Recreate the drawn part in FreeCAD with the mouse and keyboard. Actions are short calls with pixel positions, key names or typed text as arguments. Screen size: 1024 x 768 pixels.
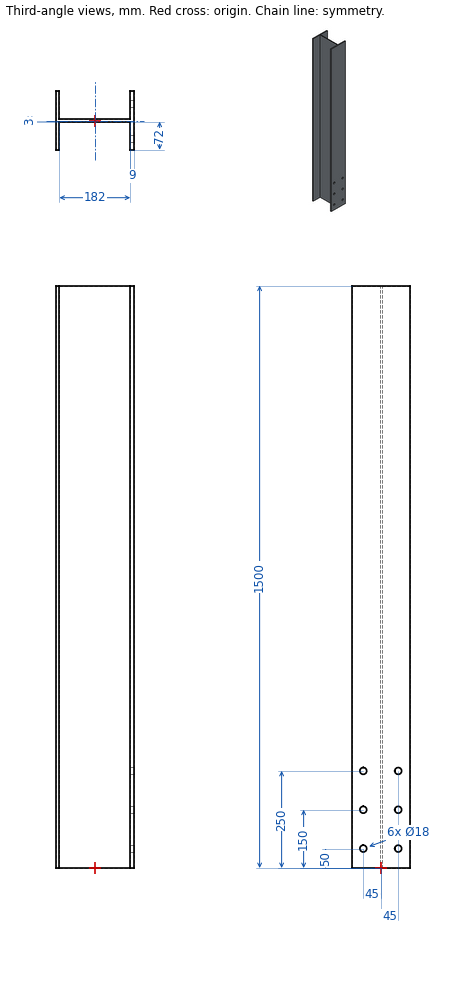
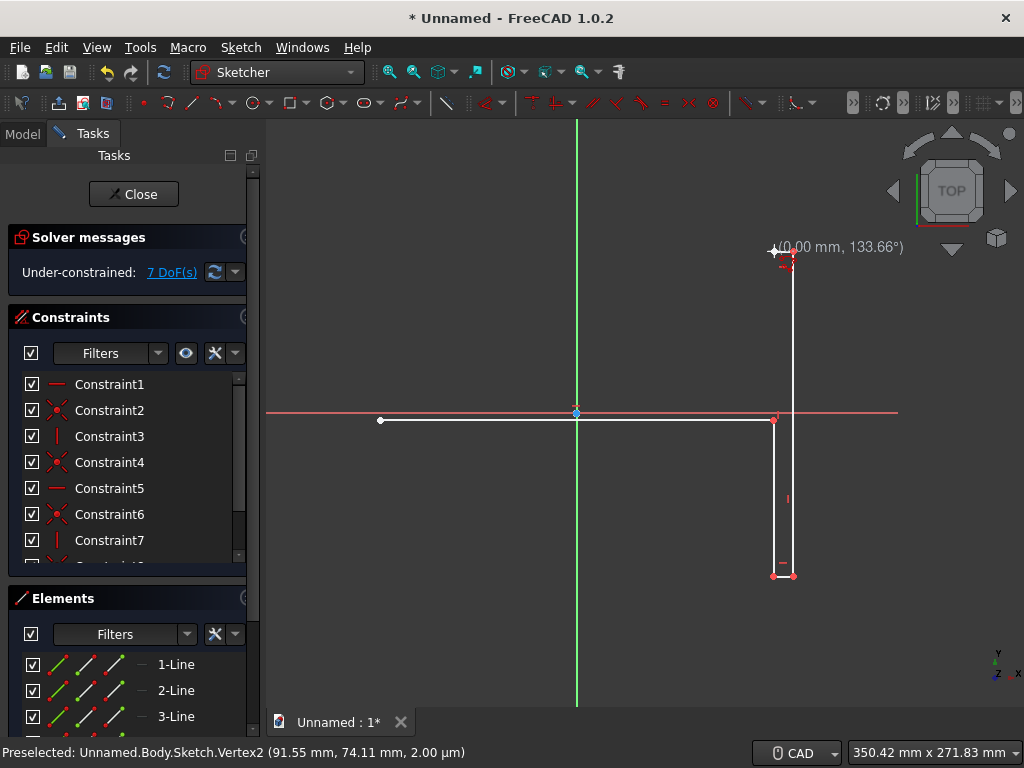
scroll(774, 407, up, 5)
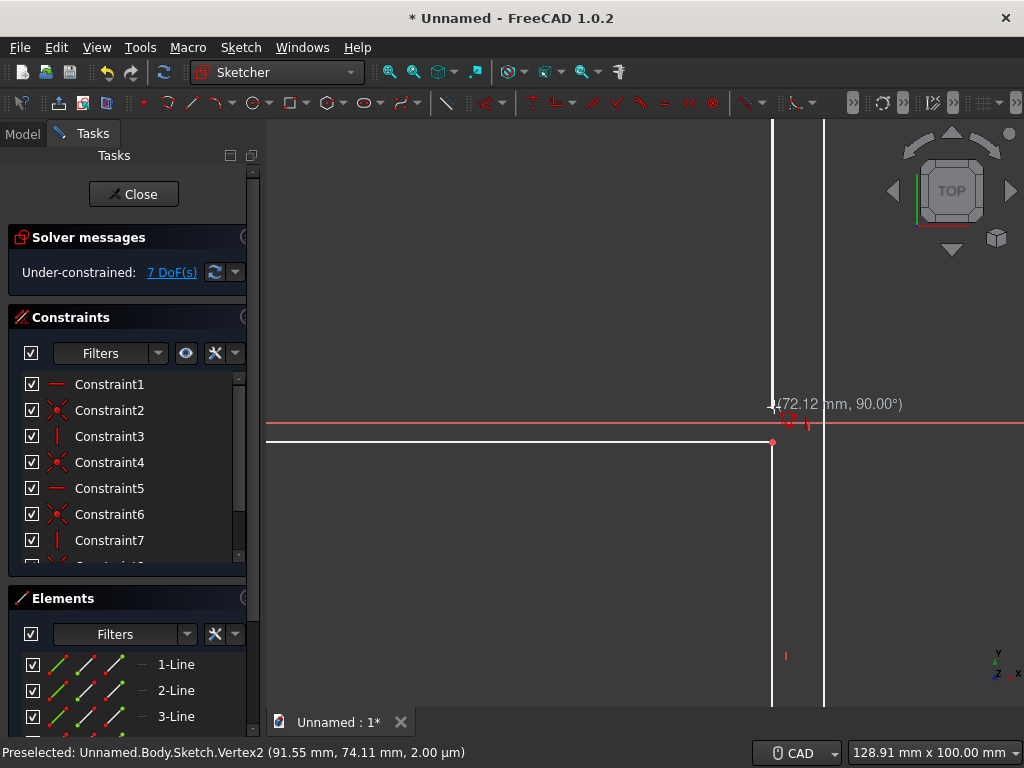
click(773, 406)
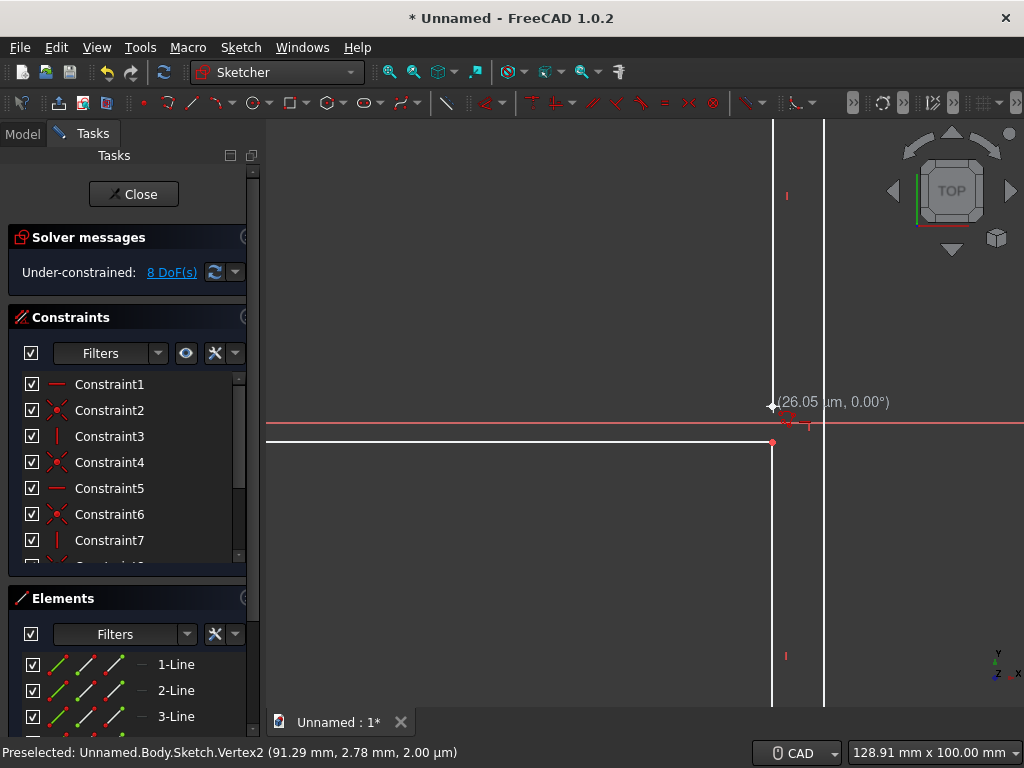
scroll(774, 407, down, 5)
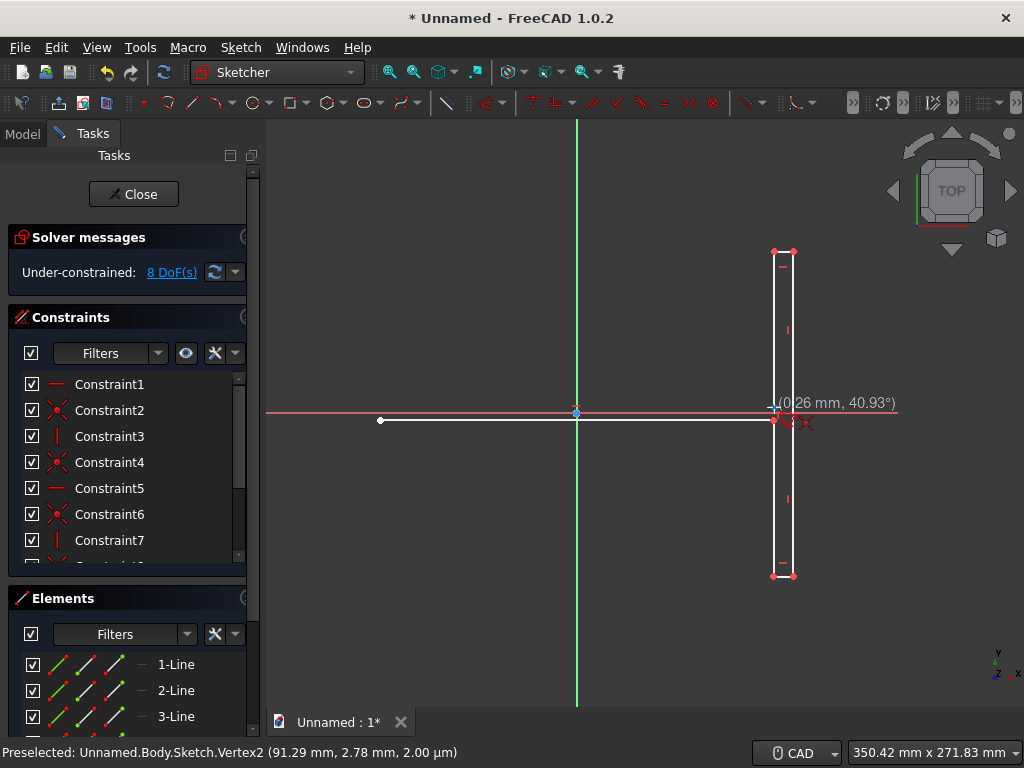
scroll(380, 407, up, 5)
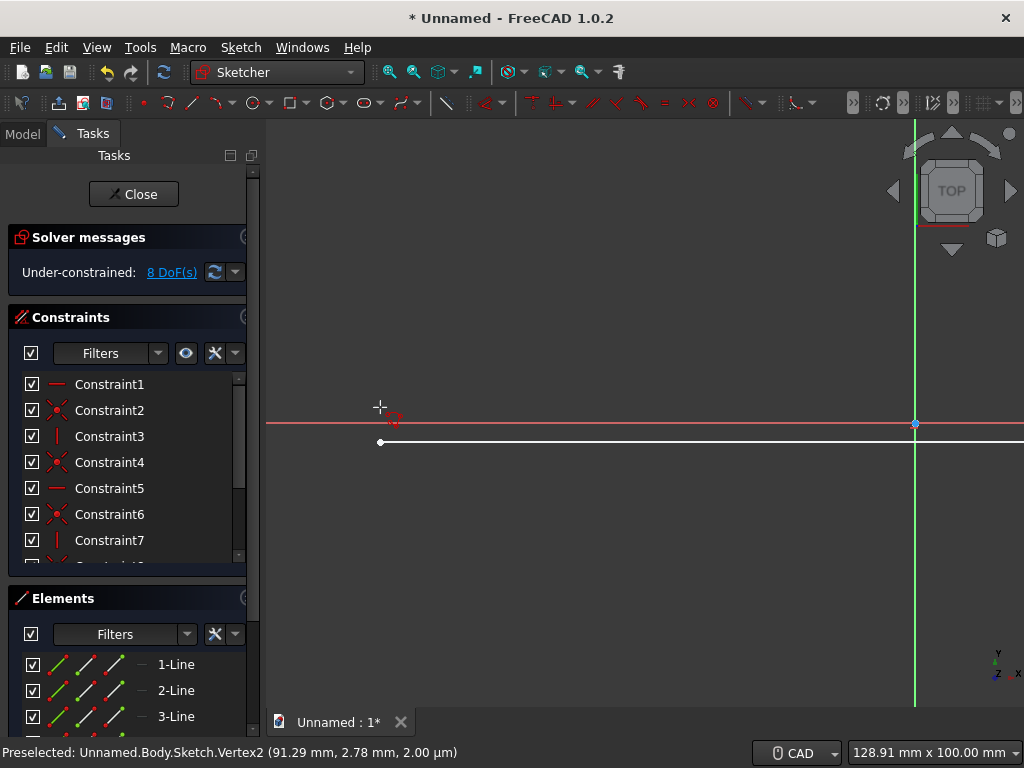
click(380, 406)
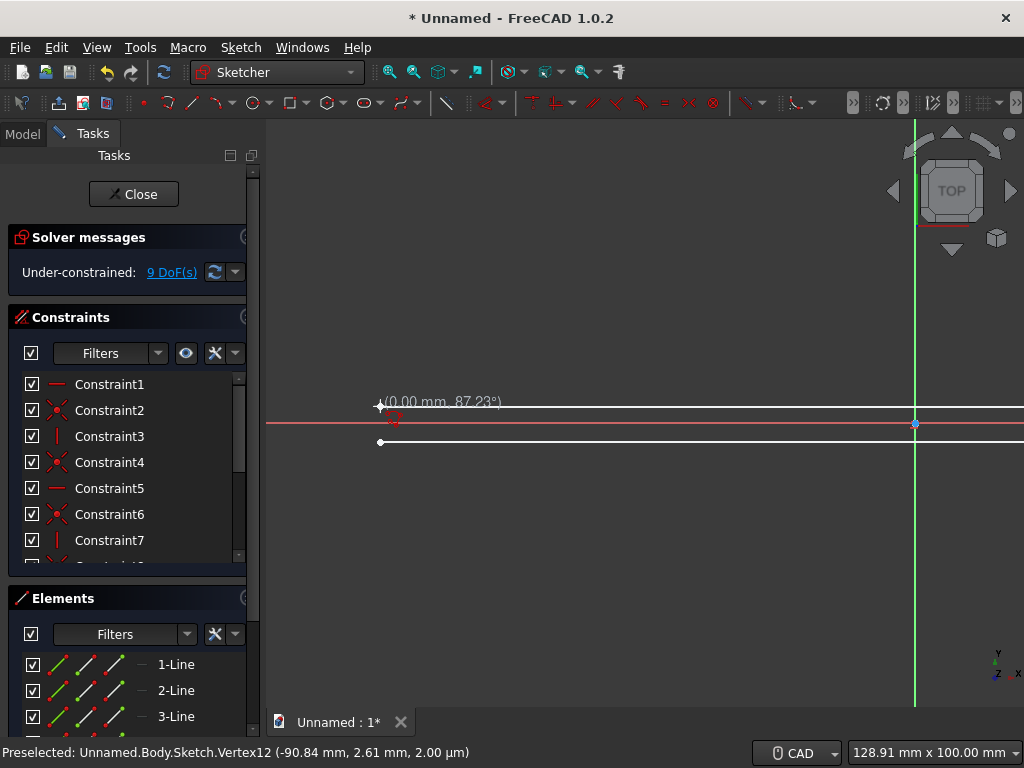
scroll(379, 407, down, 5)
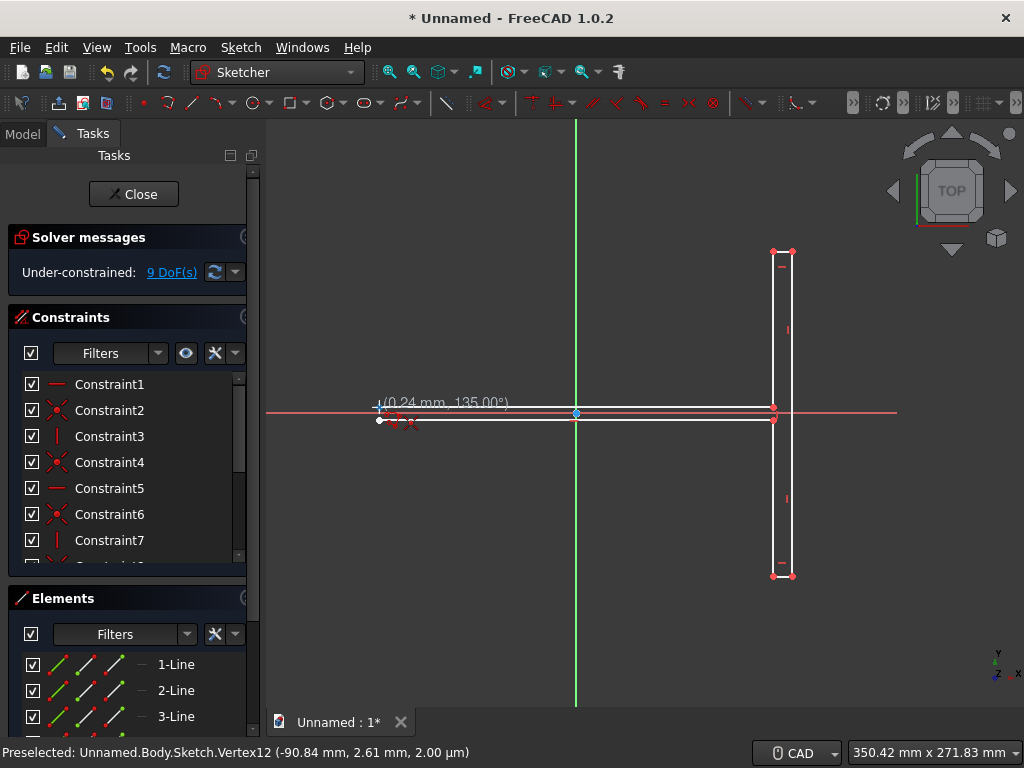
click(379, 251)
click(360, 251)
click(360, 576)
click(379, 576)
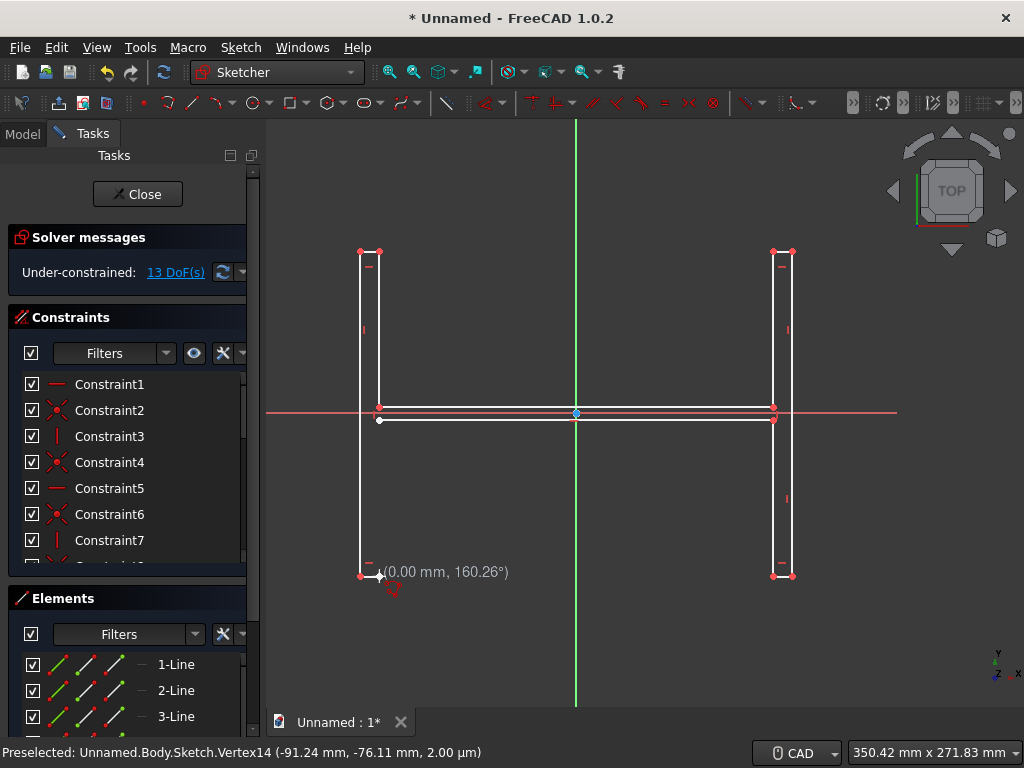
scroll(379, 420, up, 5)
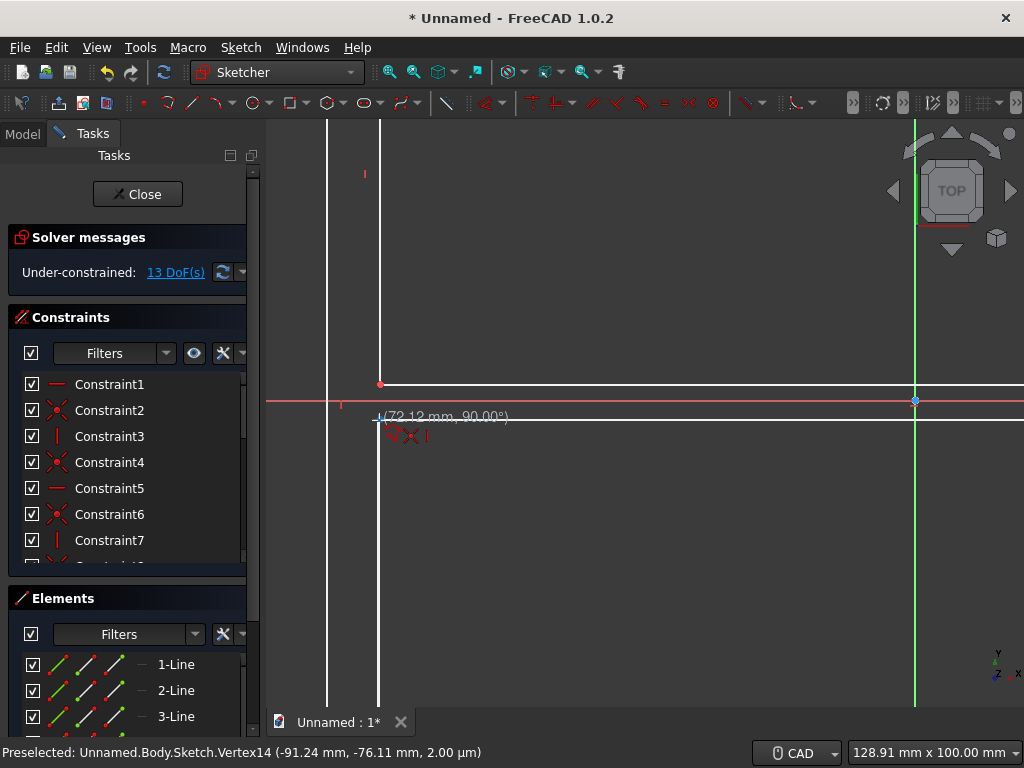
click(380, 420)
key(Escape)
key(Escape)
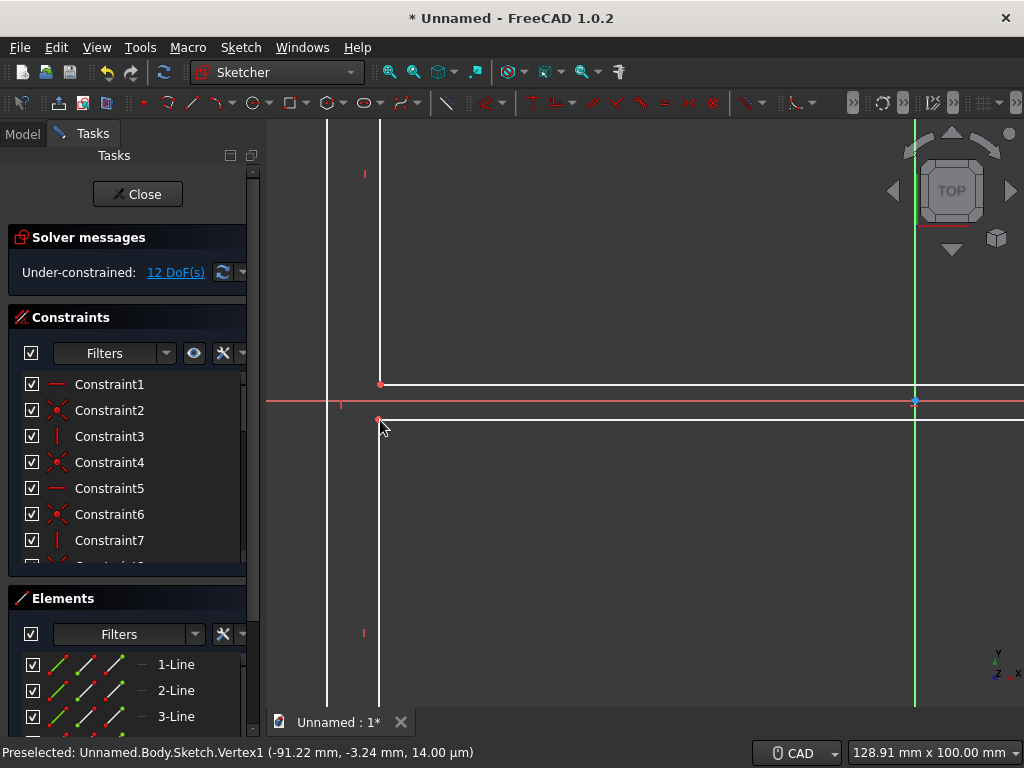
scroll(379, 420, down, 5)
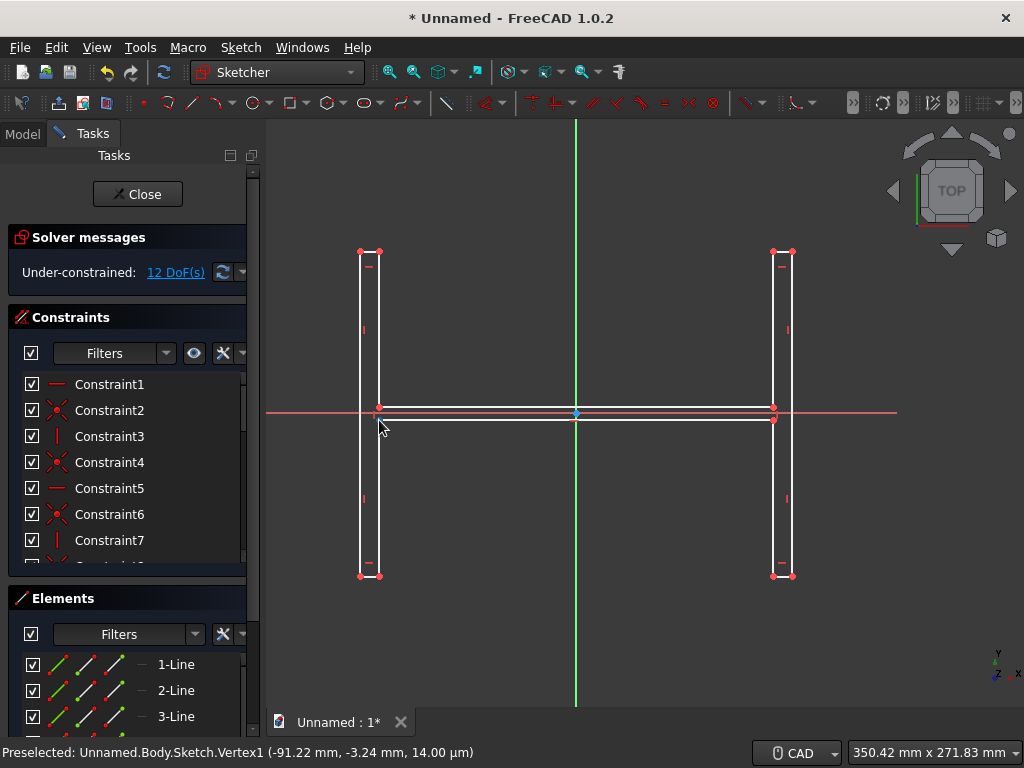
click(773, 577)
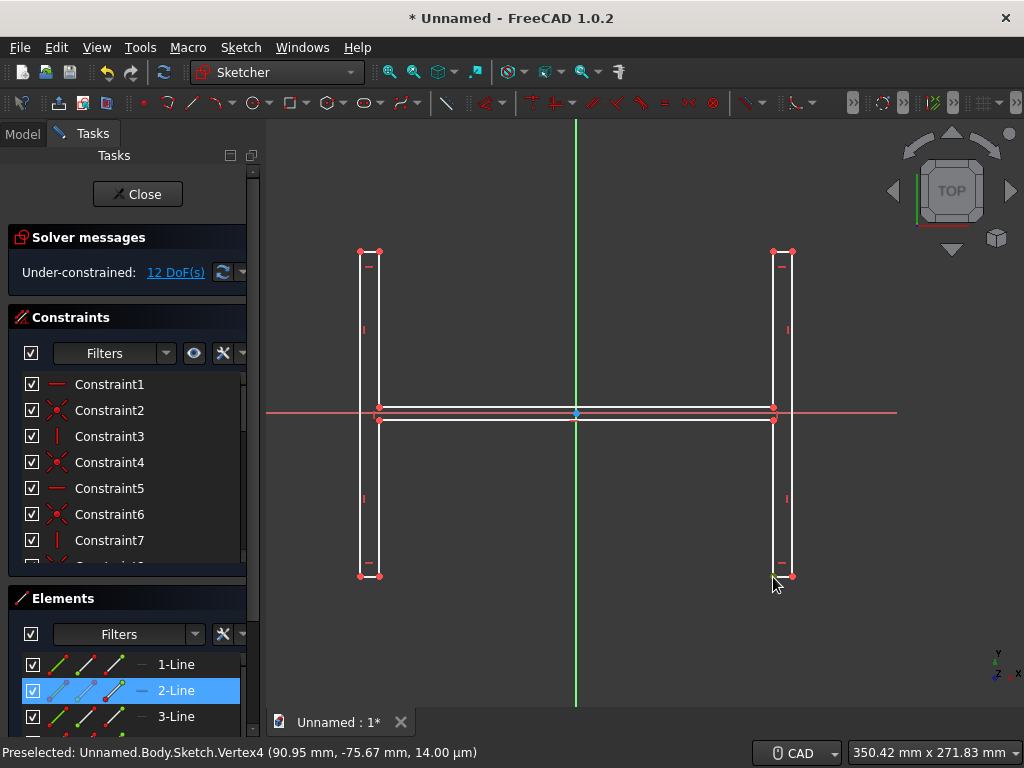
click(773, 252)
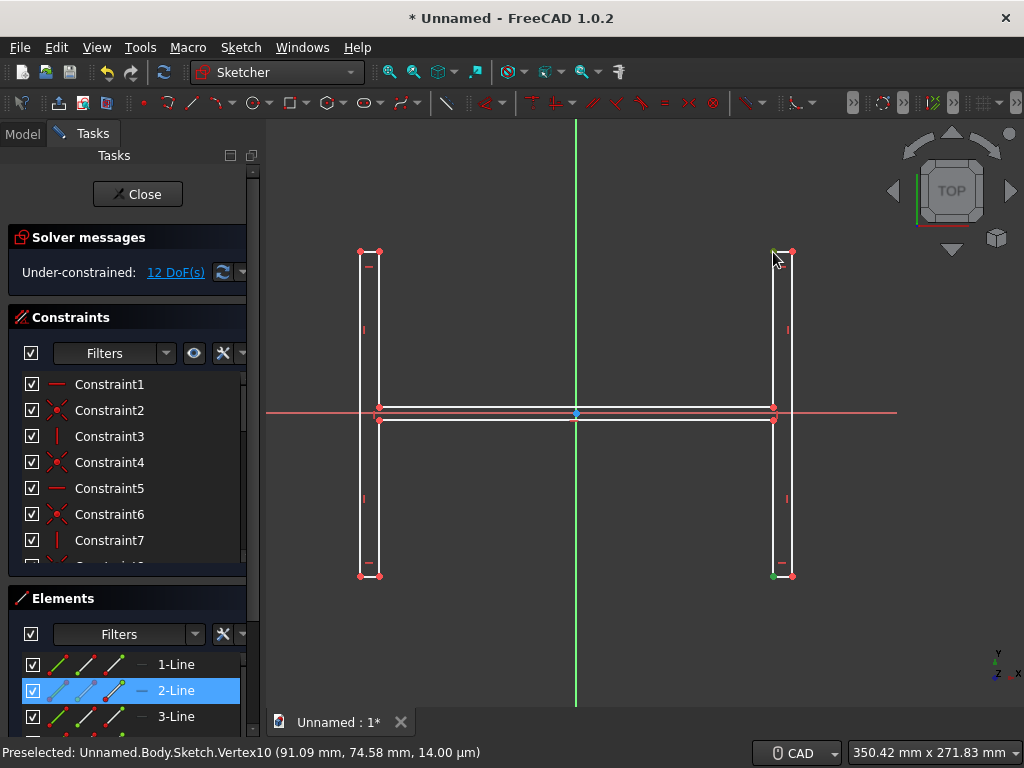
click(819, 413)